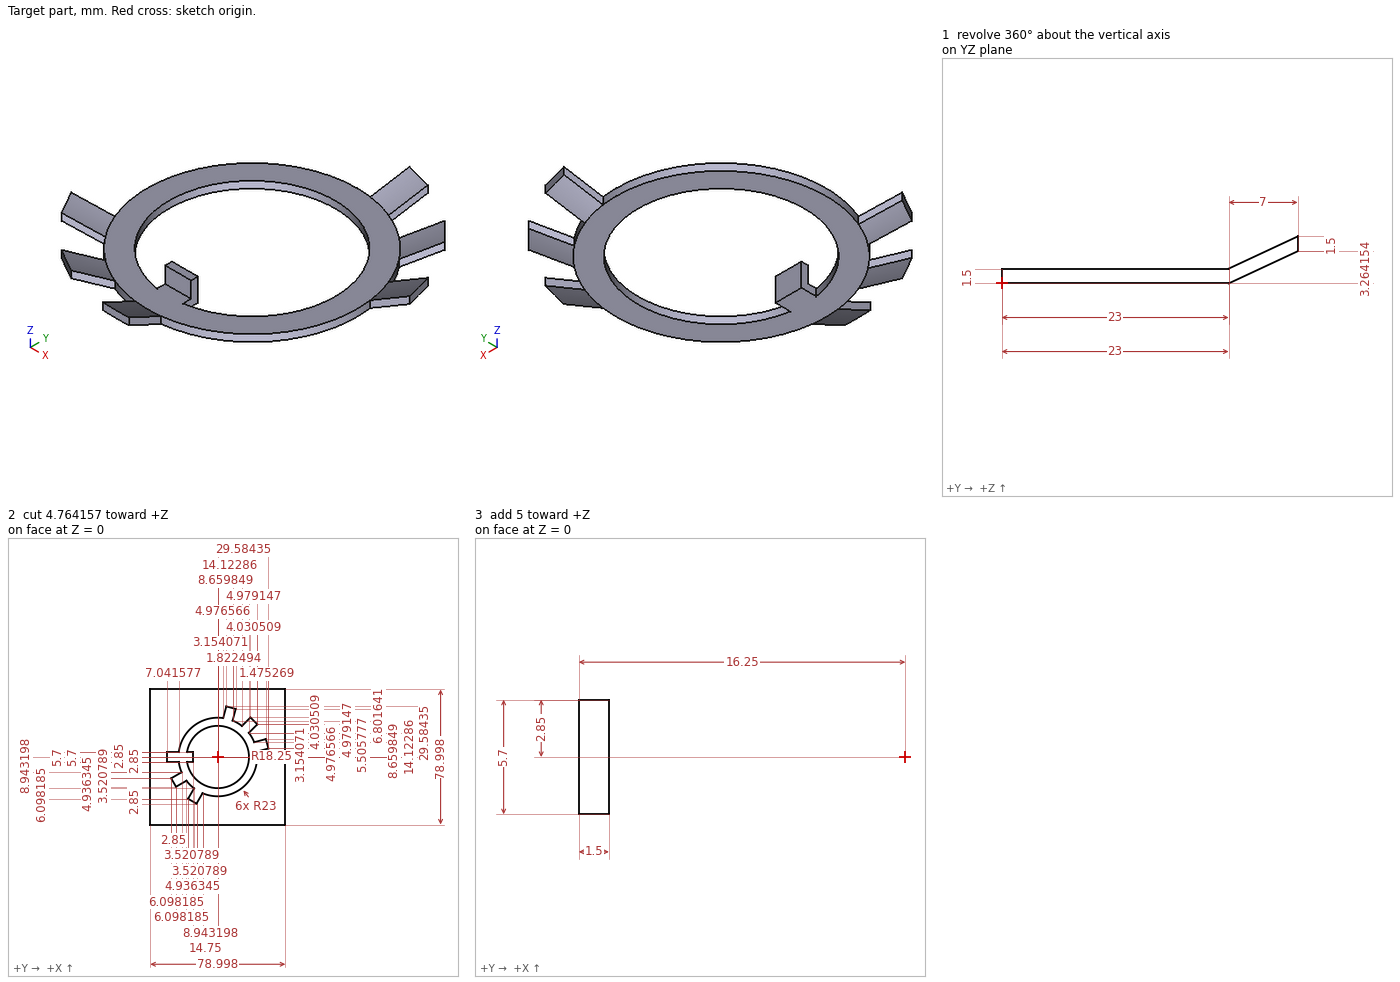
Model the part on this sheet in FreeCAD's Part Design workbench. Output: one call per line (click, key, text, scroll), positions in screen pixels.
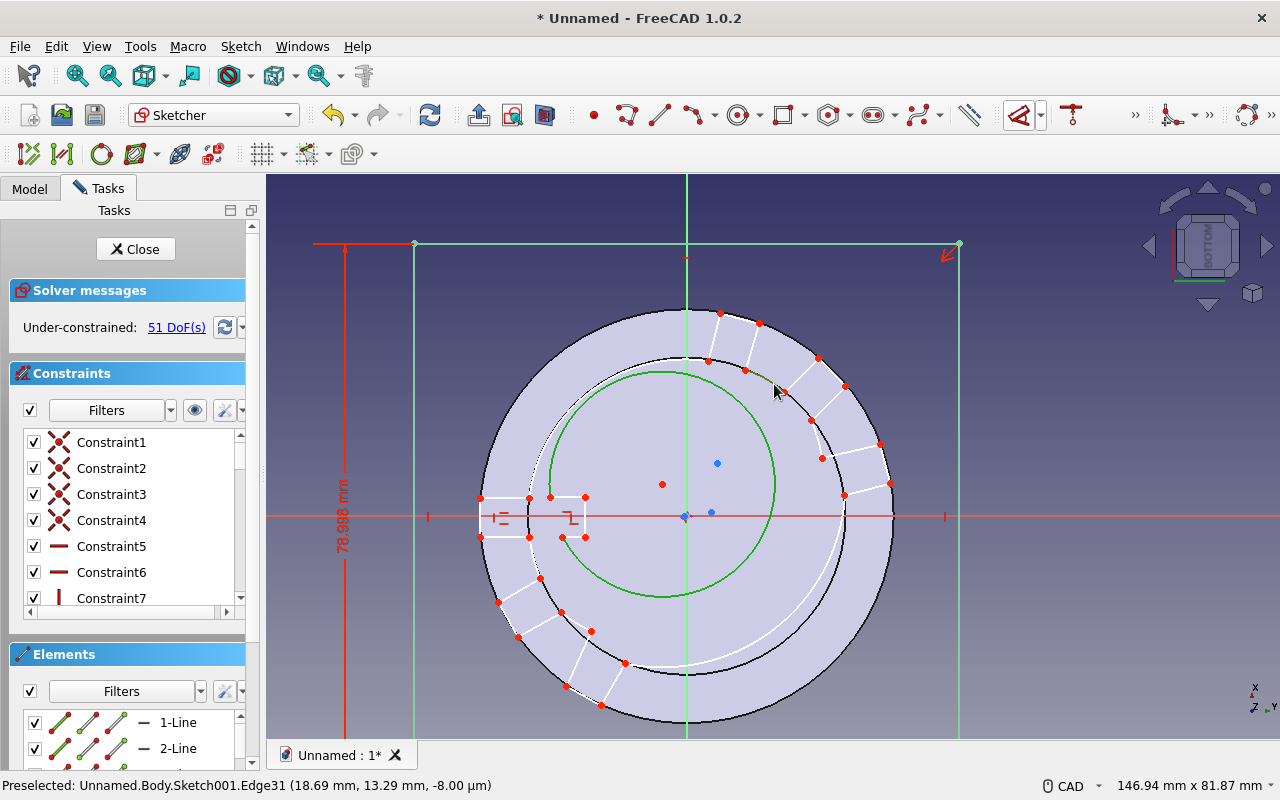
click(1071, 116)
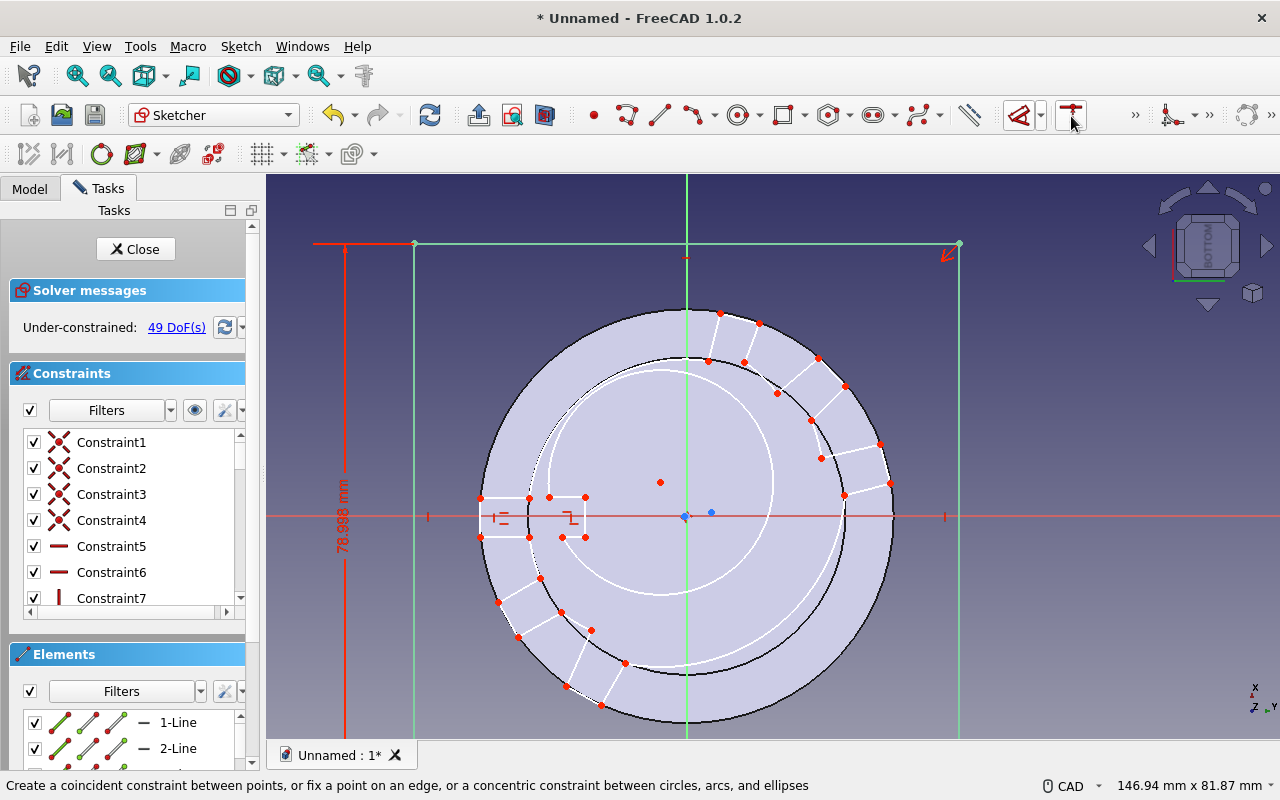
click(734, 568)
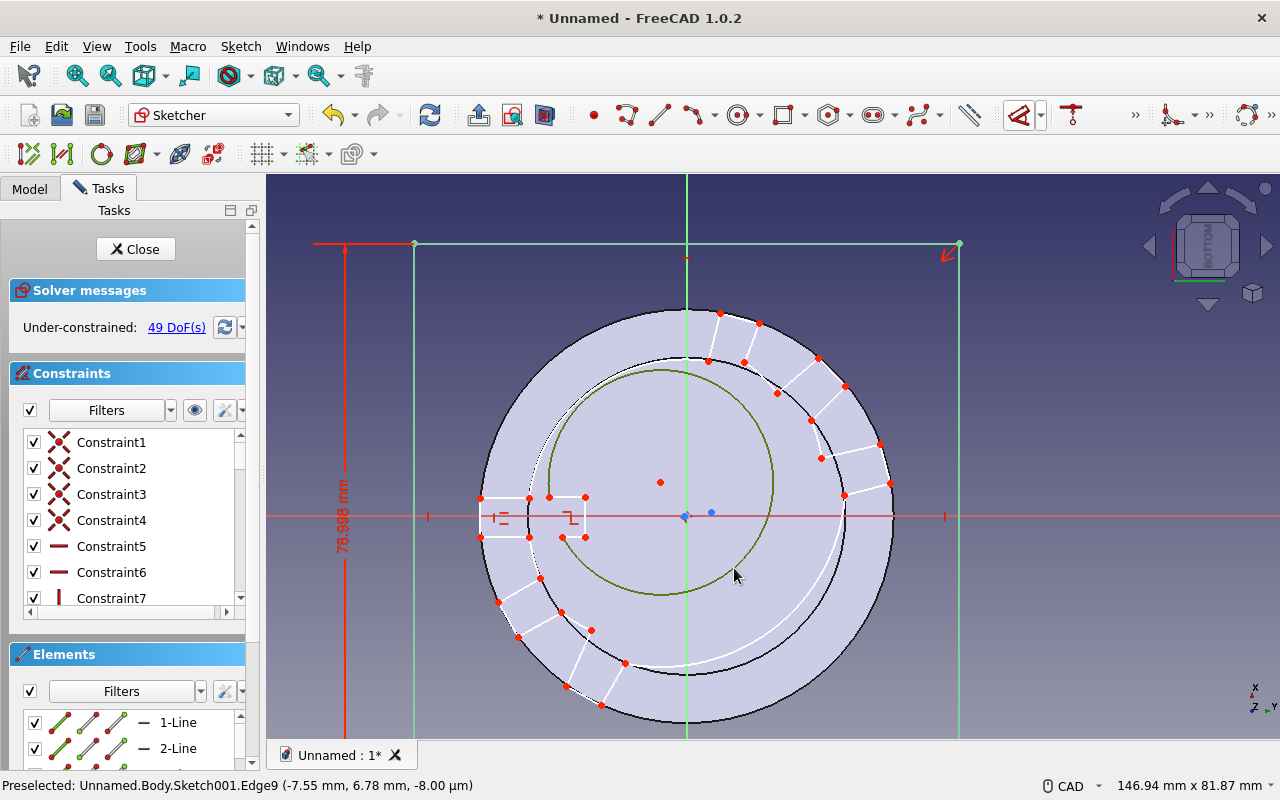
scroll(543, 450, up, 2)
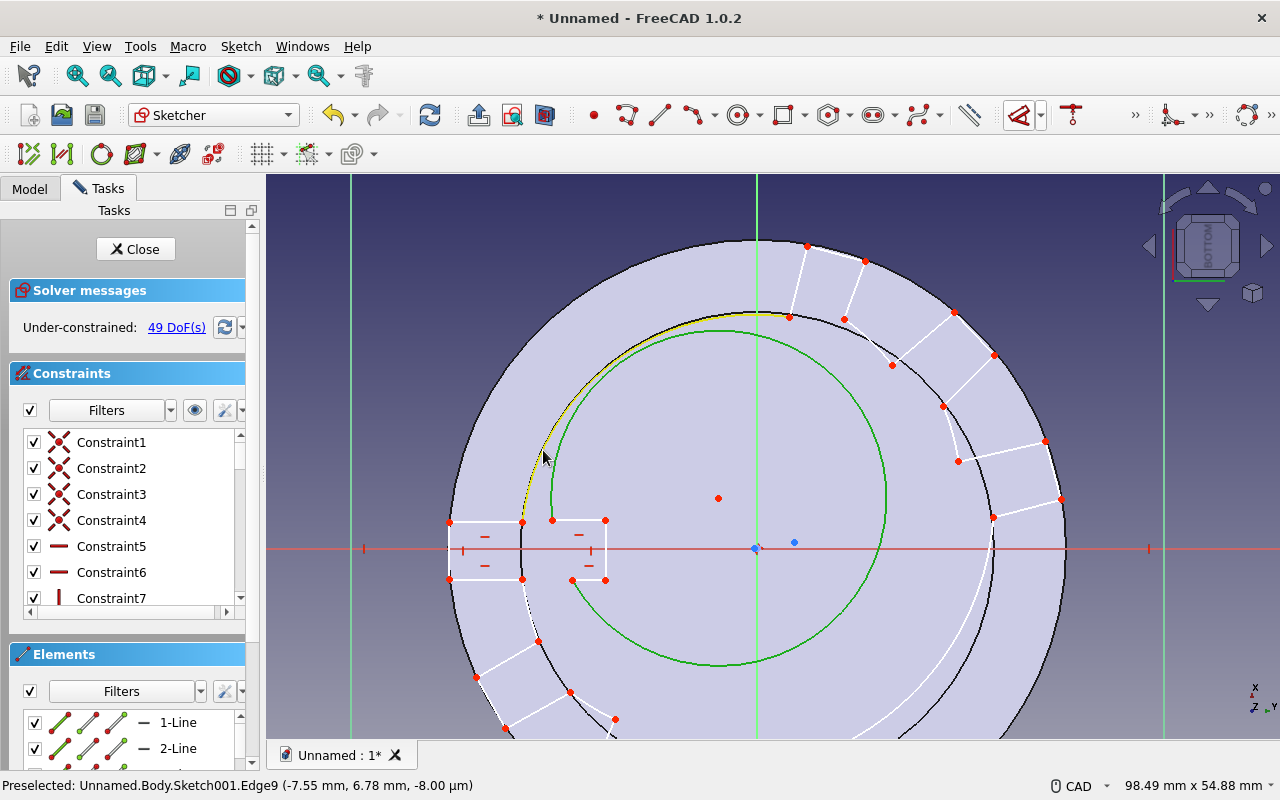
click(543, 450)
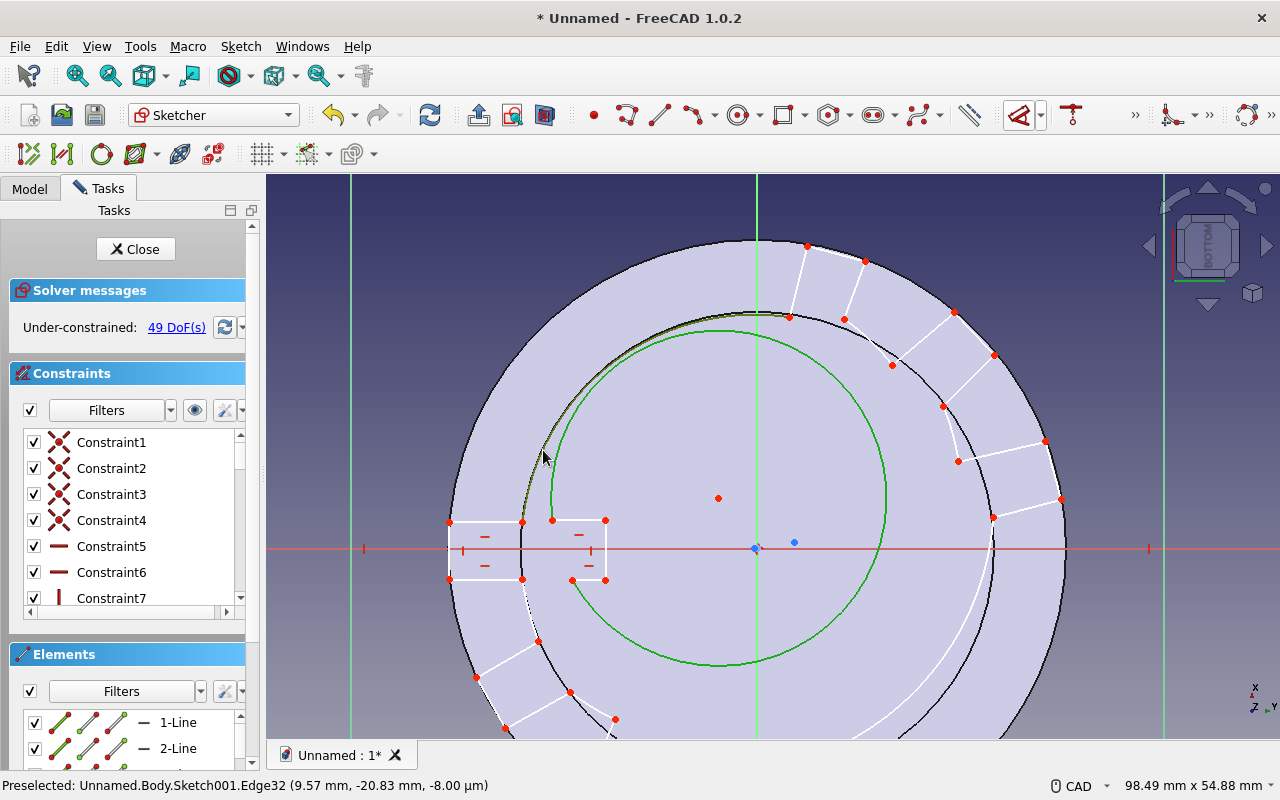
key(c)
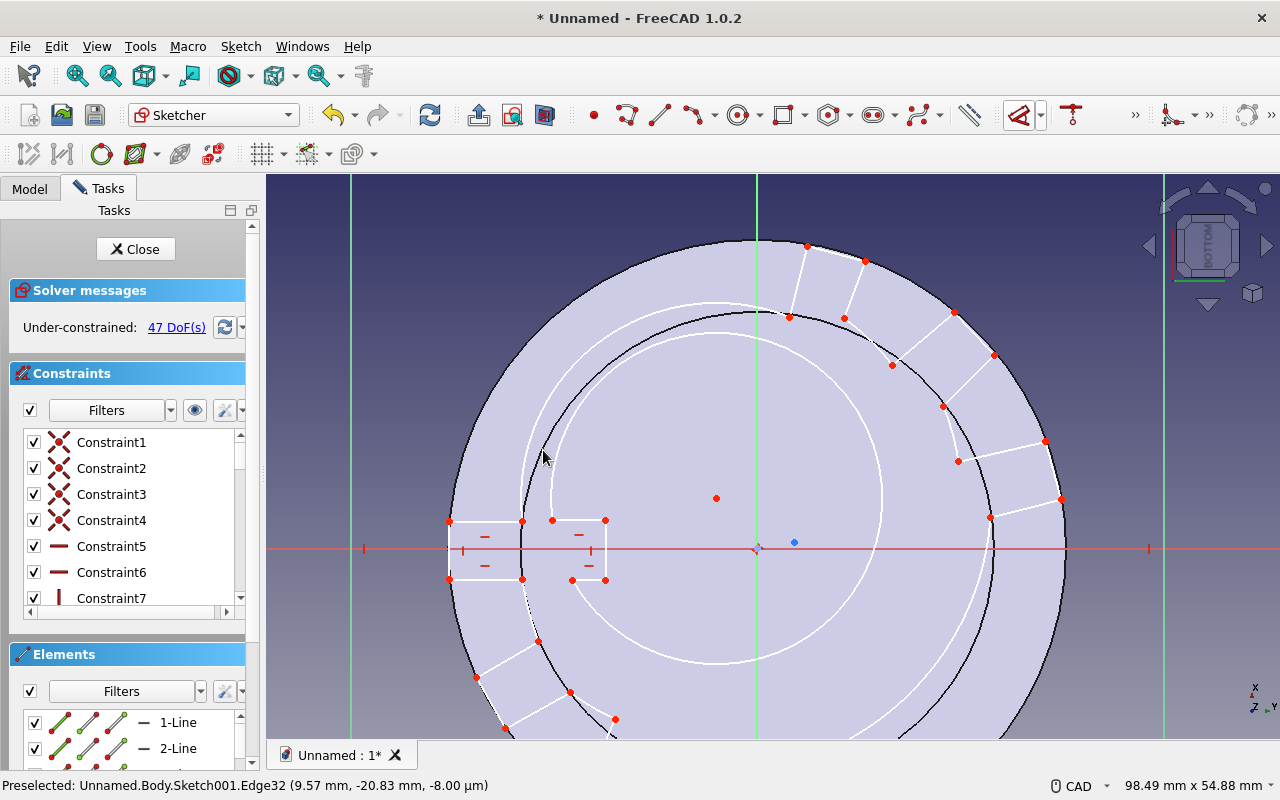
click(825, 624)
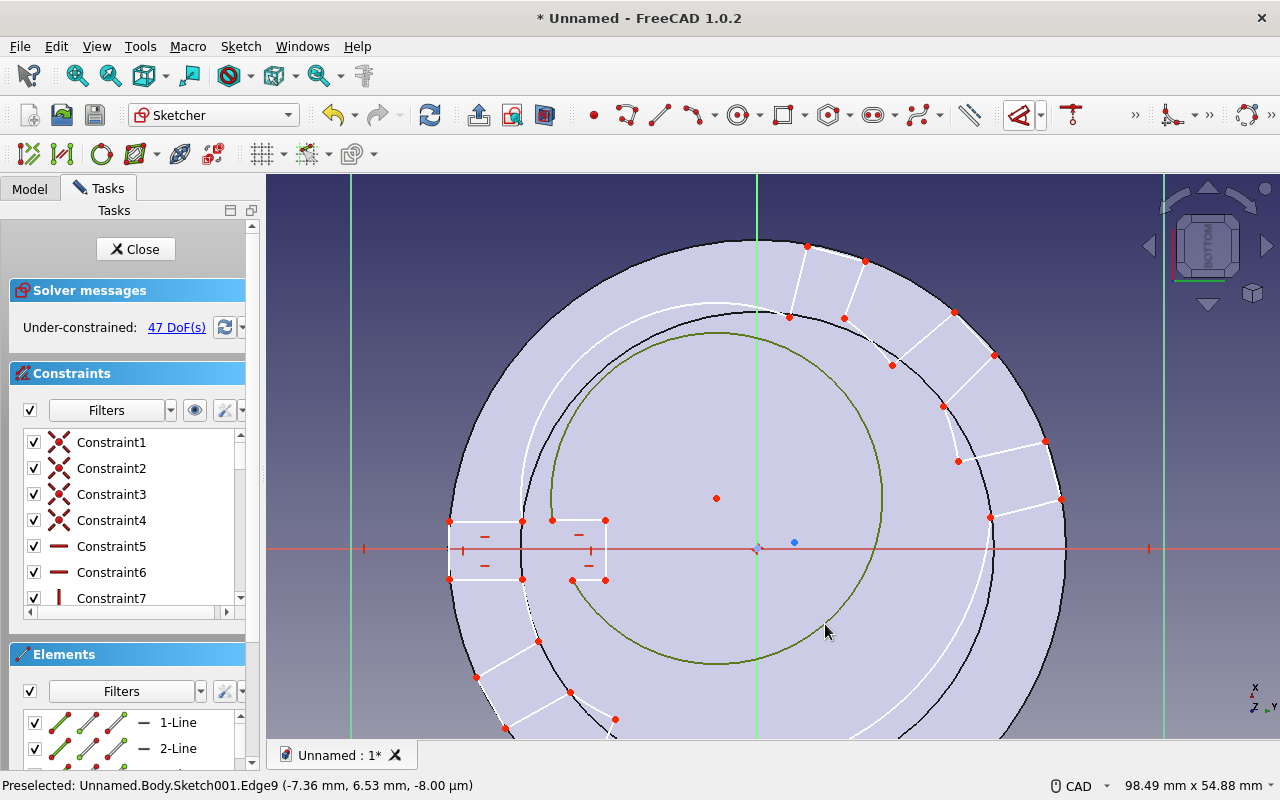
click(526, 599)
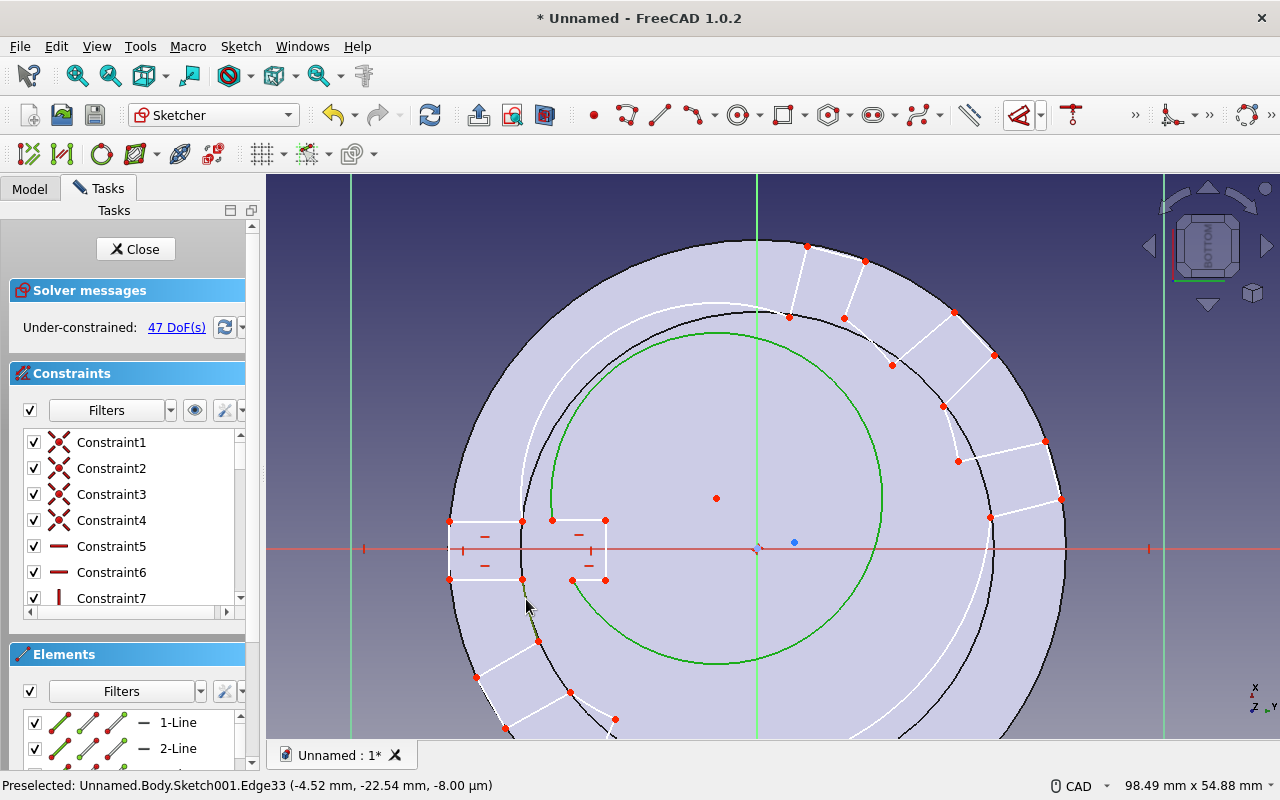
key(c)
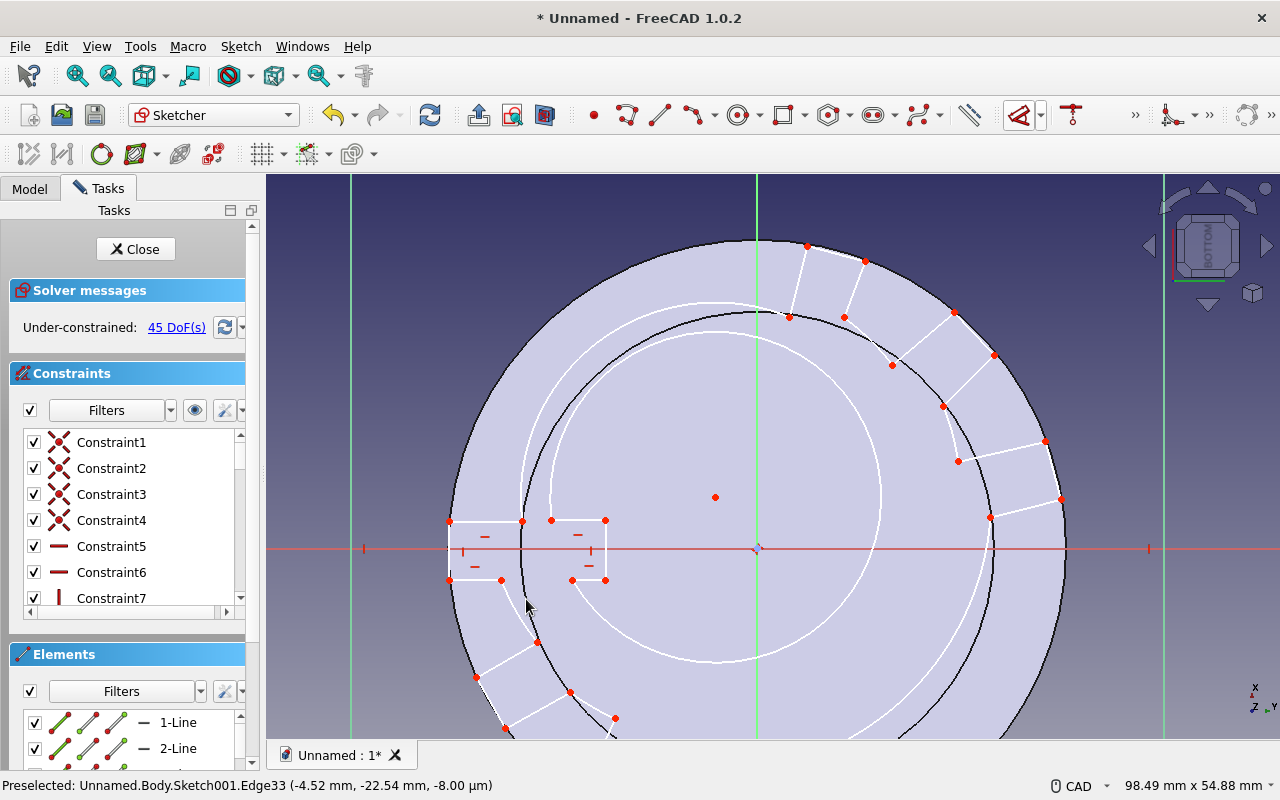
drag(706, 487, 767, 559)